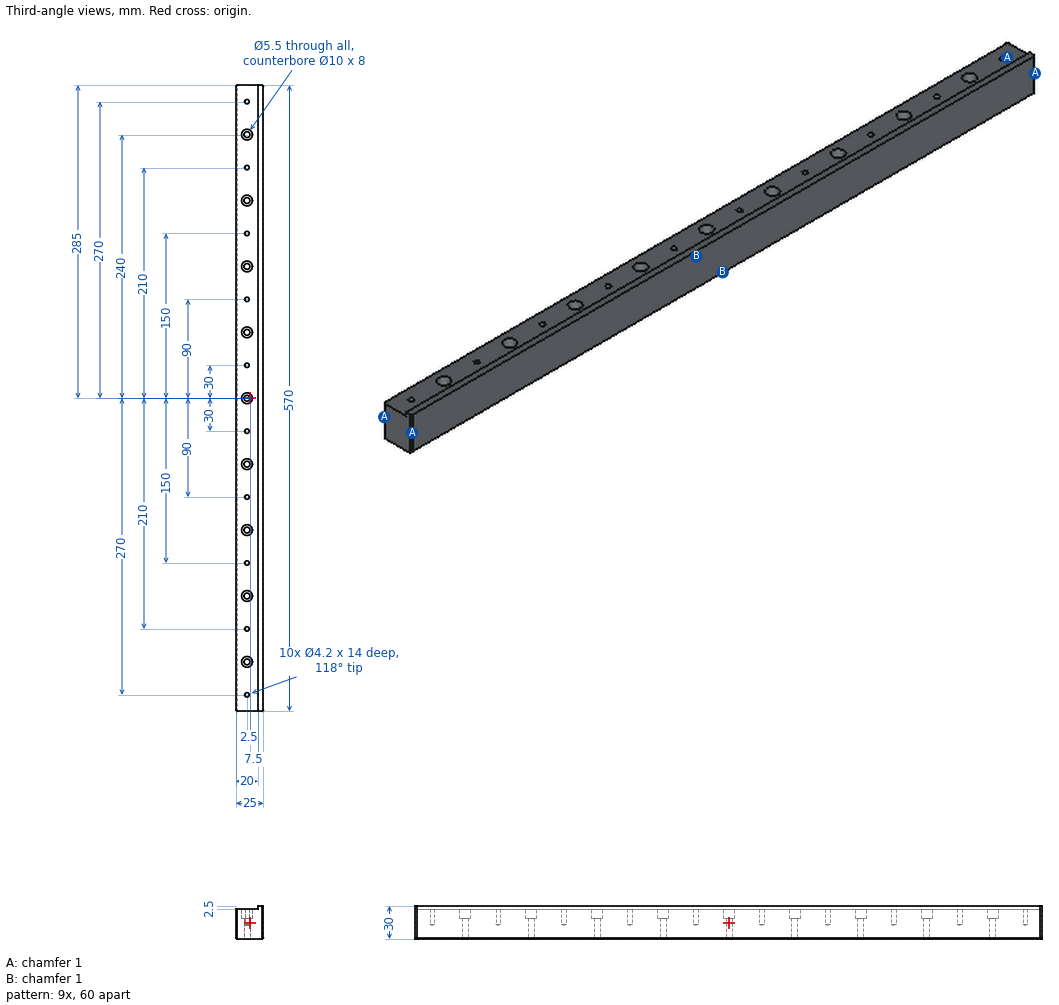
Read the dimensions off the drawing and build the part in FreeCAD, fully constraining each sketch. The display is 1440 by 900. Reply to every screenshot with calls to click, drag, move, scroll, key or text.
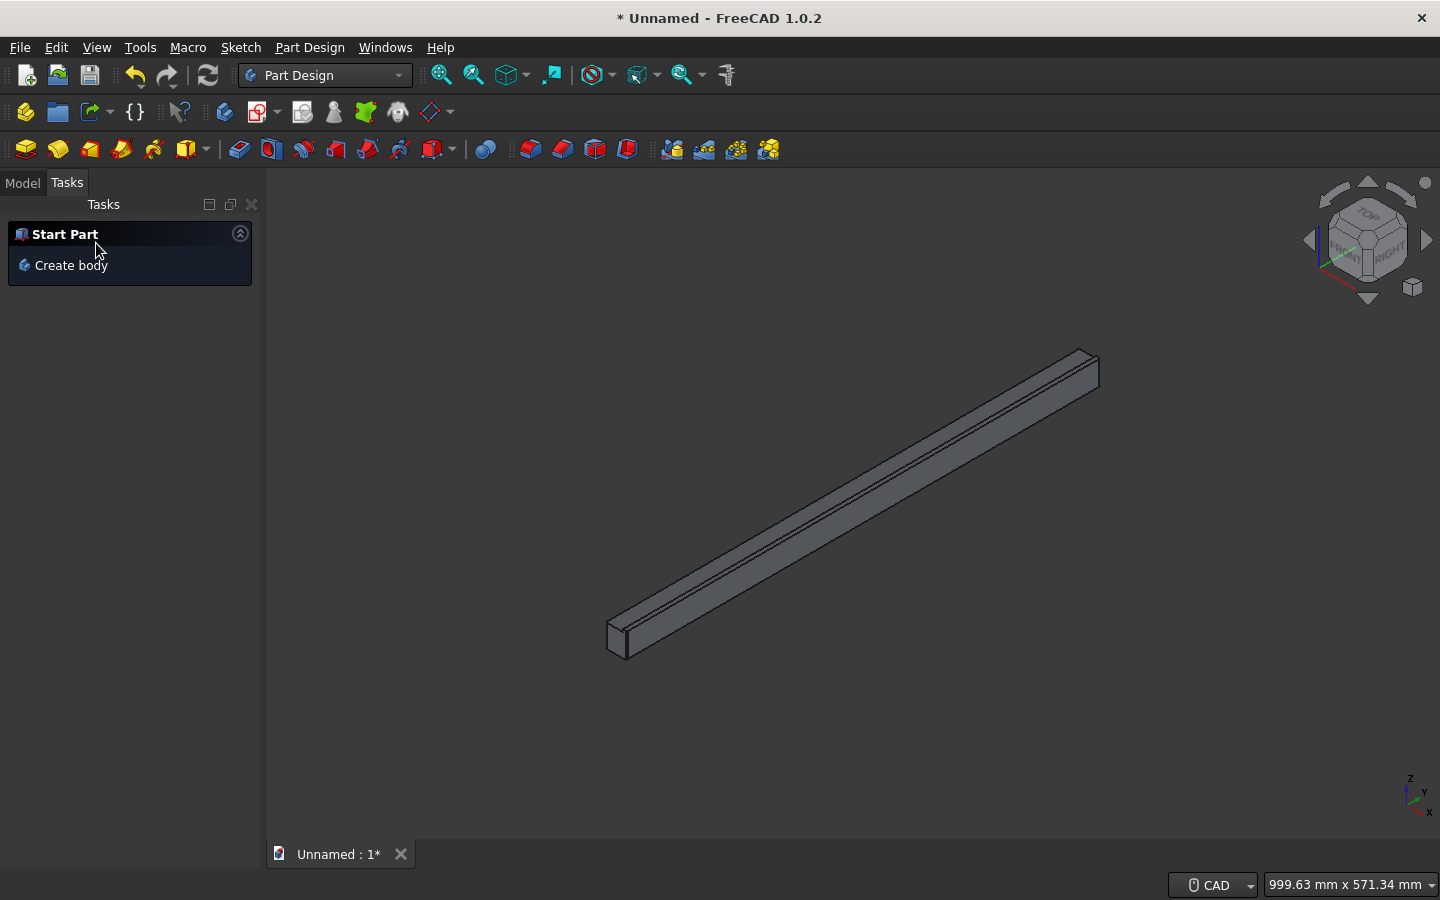
key(2)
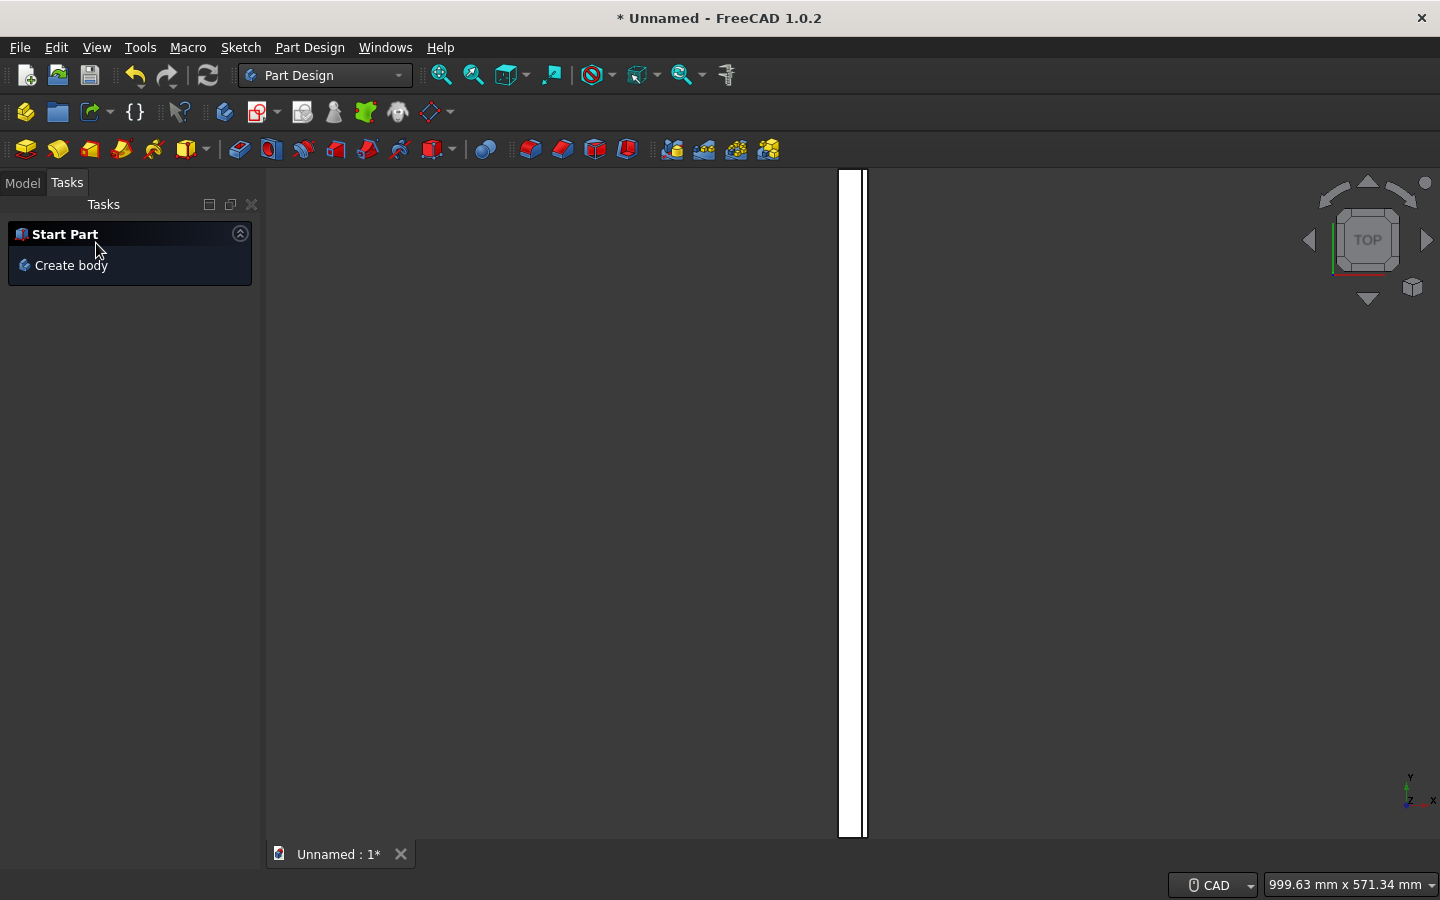
click(850, 216)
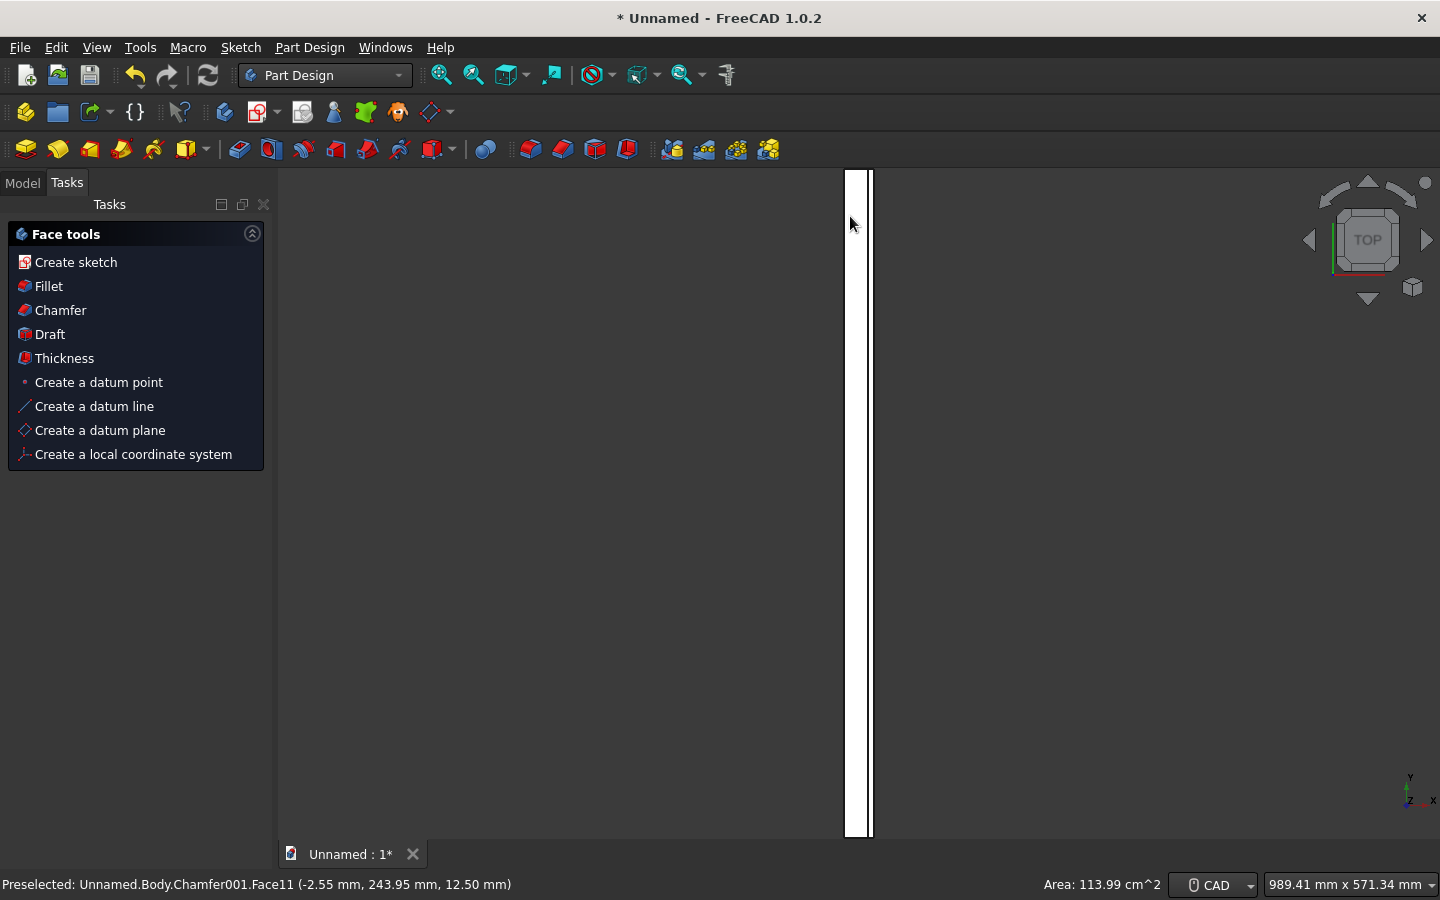
click(258, 112)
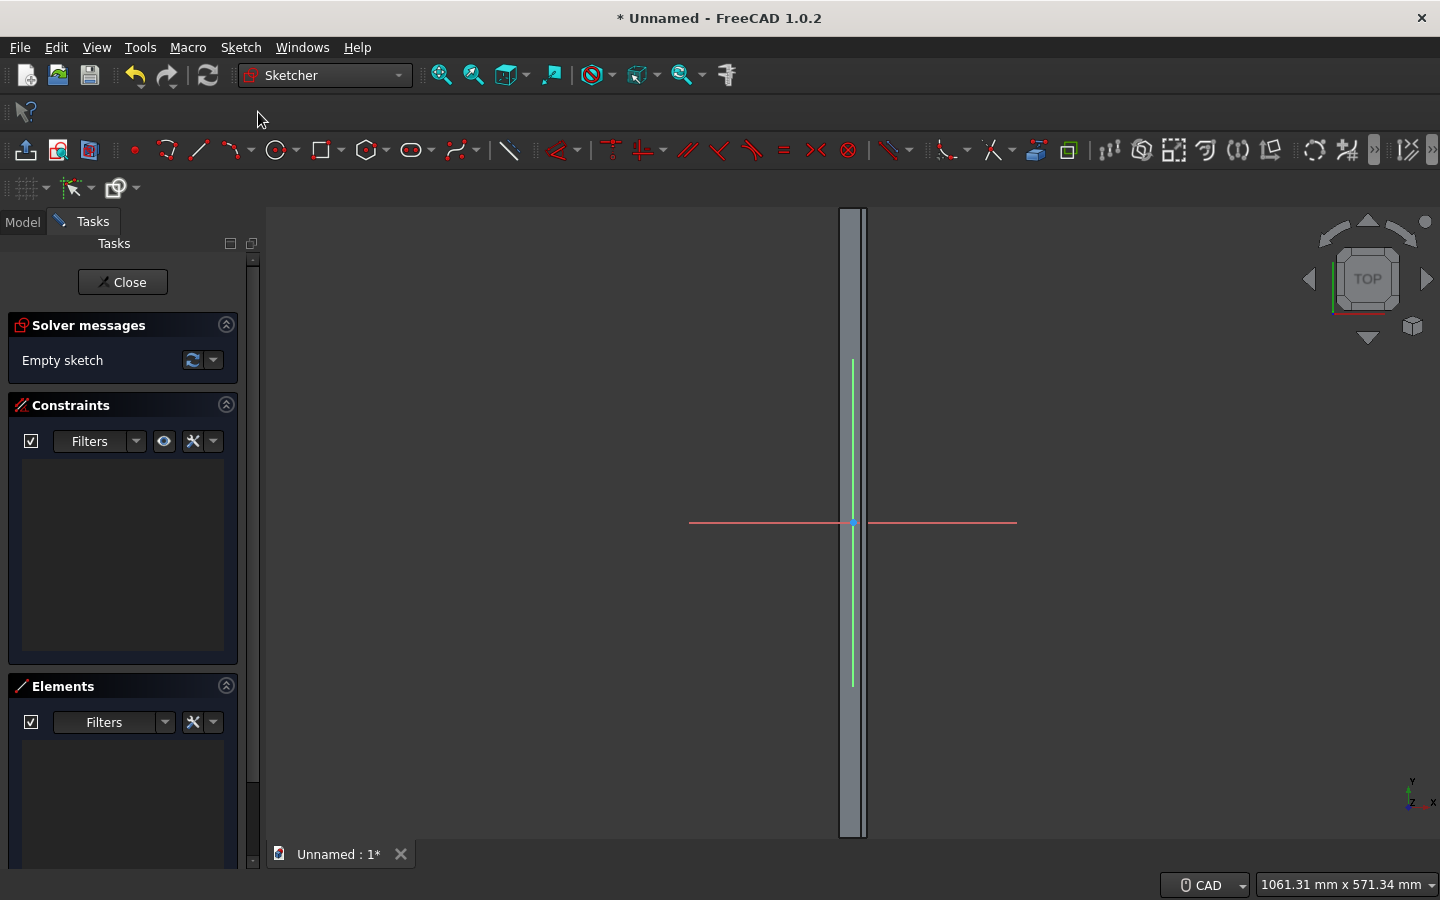
scroll(650, 523, down, 2)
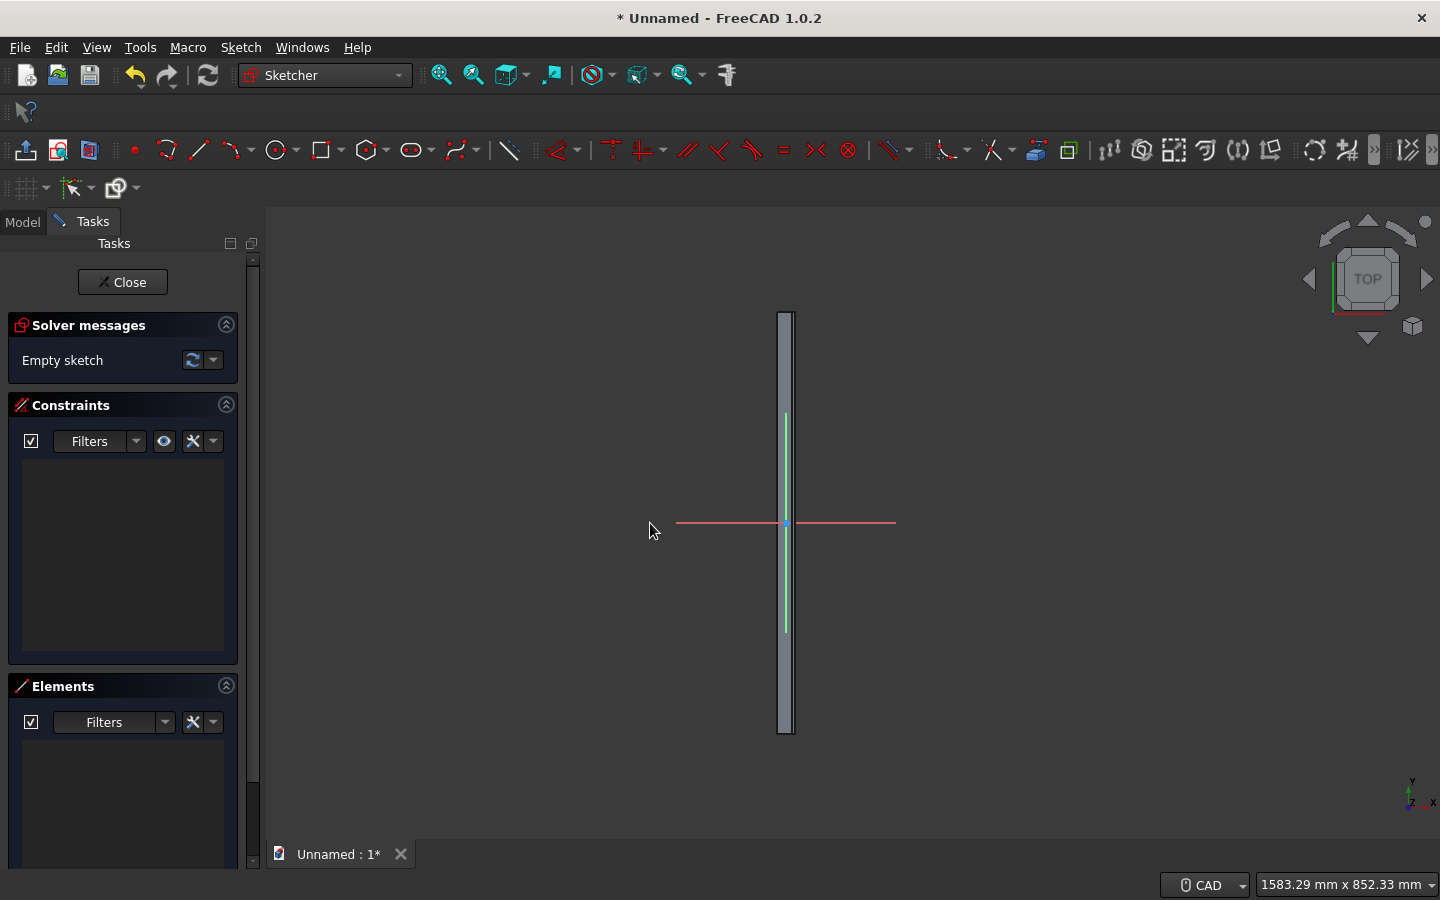
key(g)
key(c)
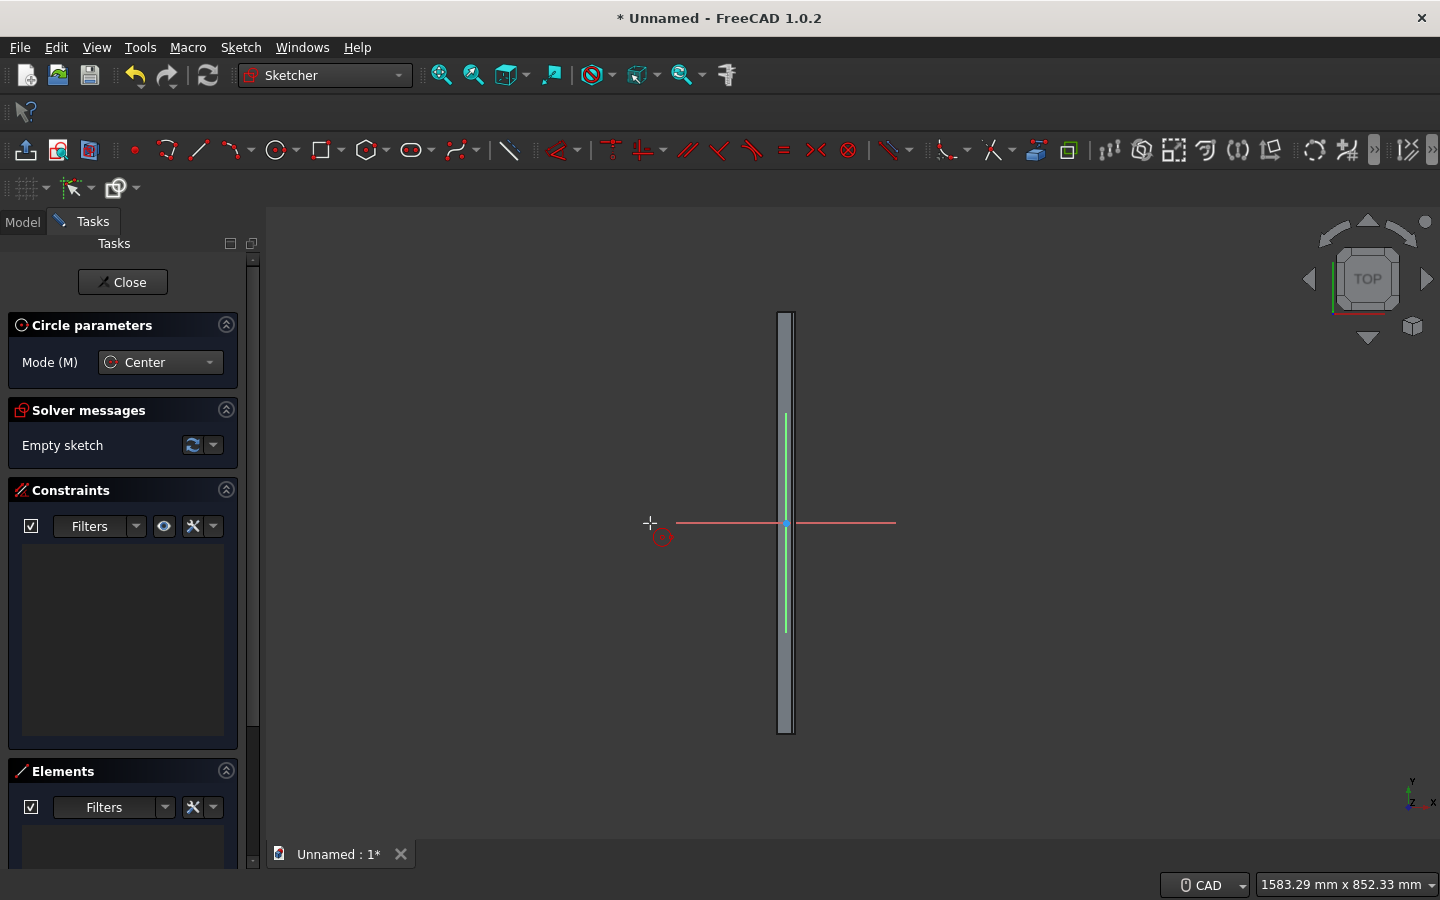
scroll(784, 723, up, 14)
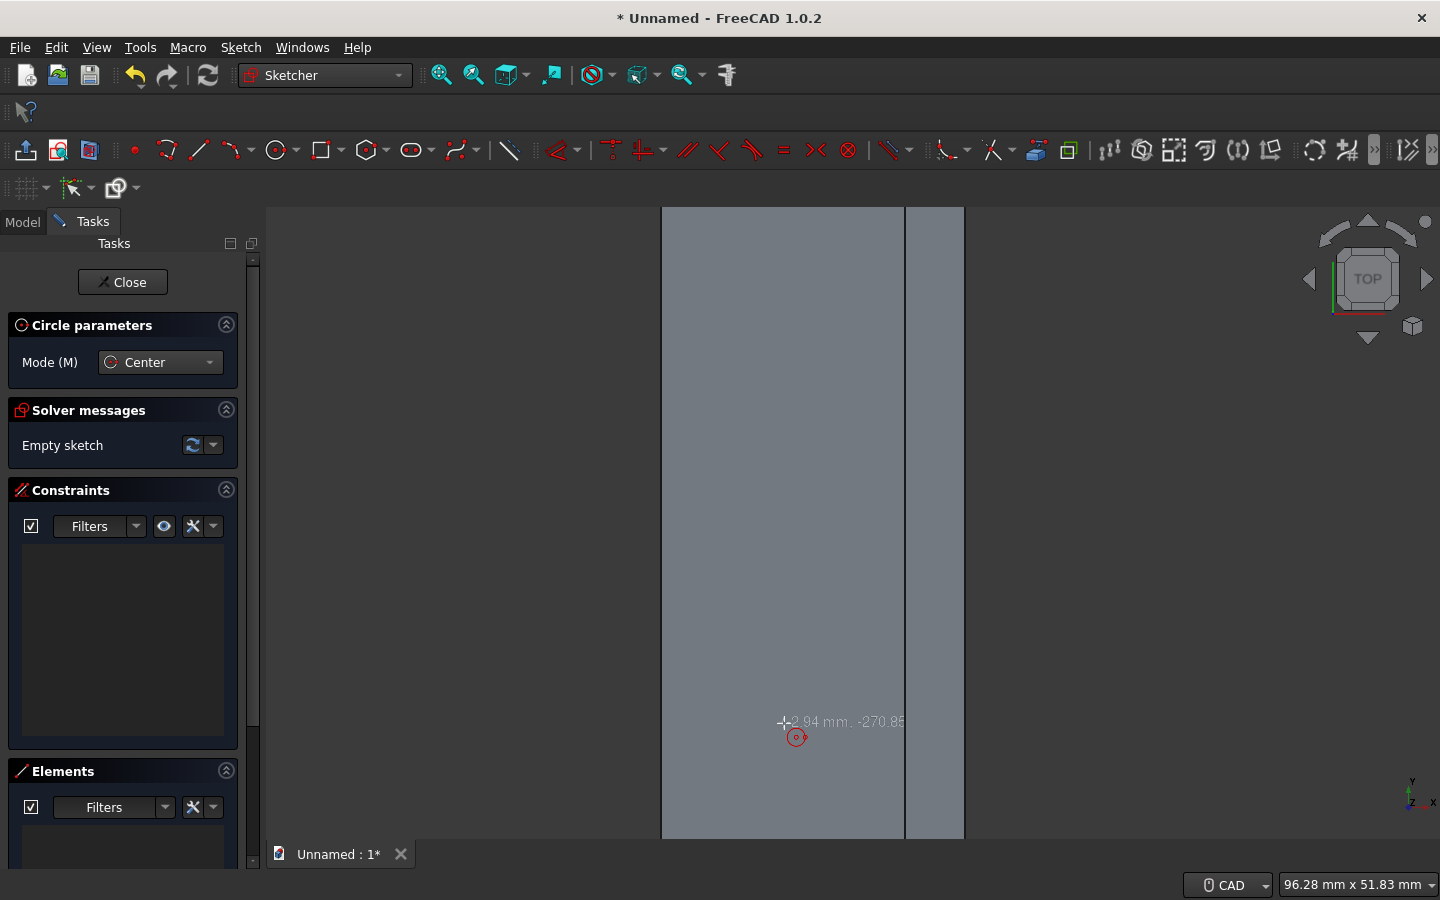
click(783, 716)